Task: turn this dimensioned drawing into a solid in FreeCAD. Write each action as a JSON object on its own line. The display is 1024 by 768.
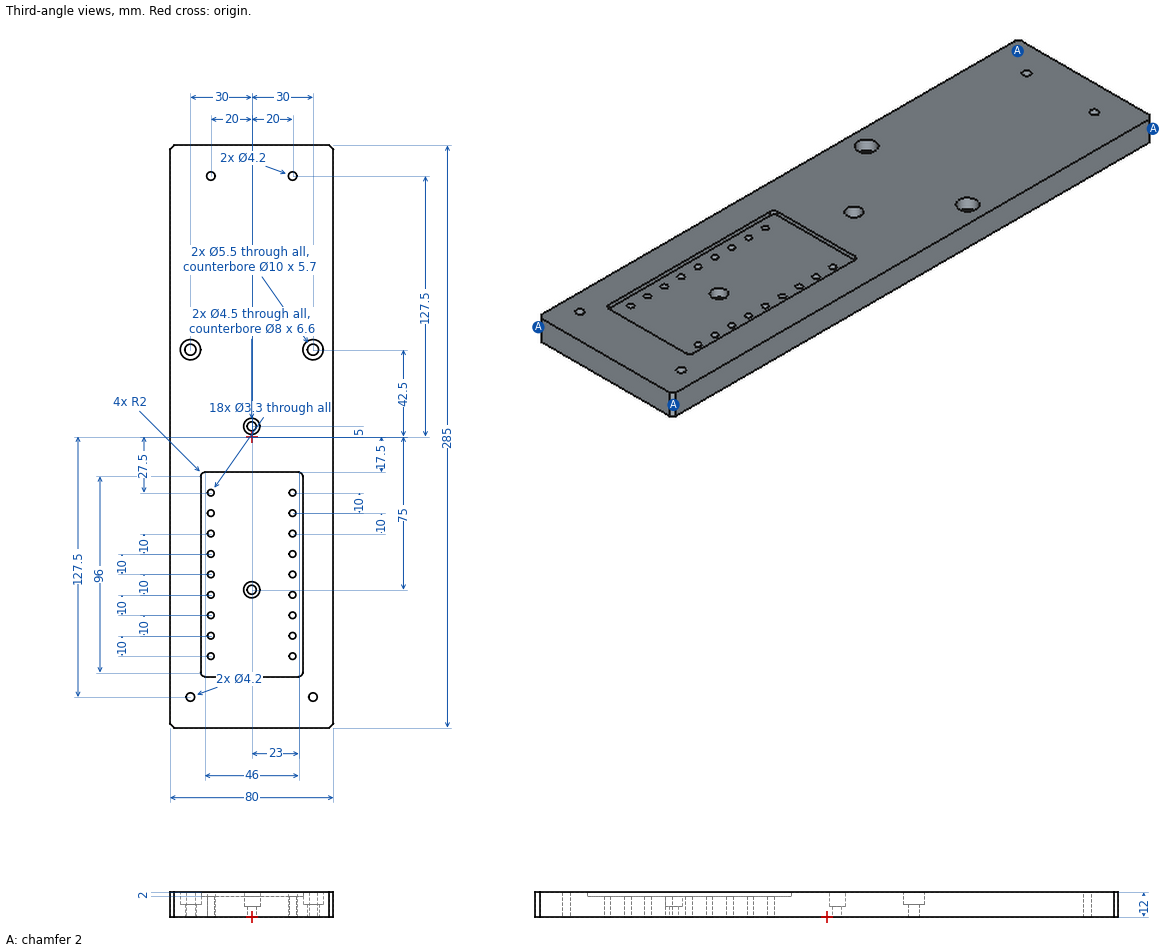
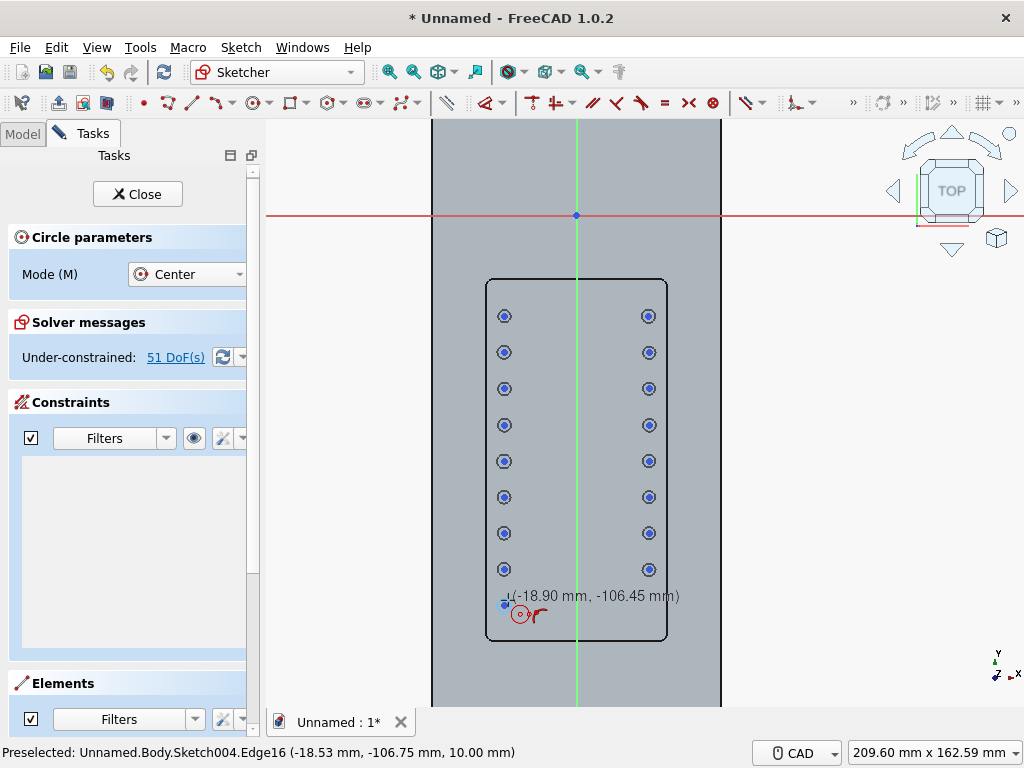
{"action": "scroll", "coordinate": [649, 605], "scroll_direction": "up", "scroll_amount": 7}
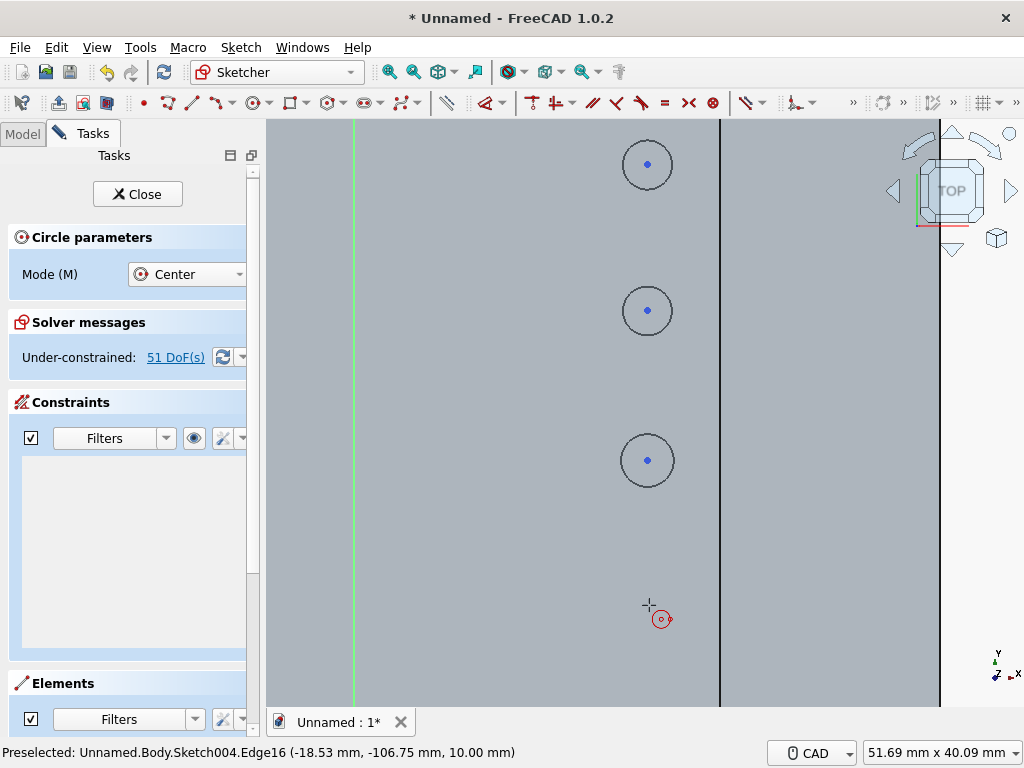
{"action": "scroll", "coordinate": [649, 605], "scroll_direction": "down", "scroll_amount": 7}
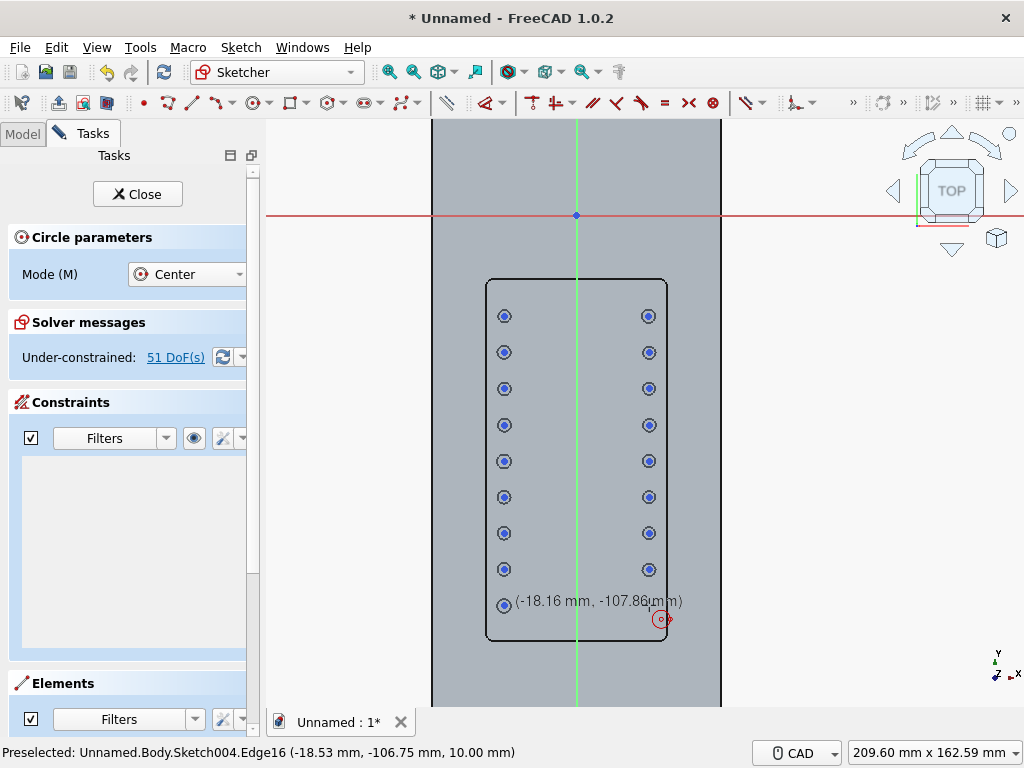
{"action": "left_click", "coordinate": [649, 605]}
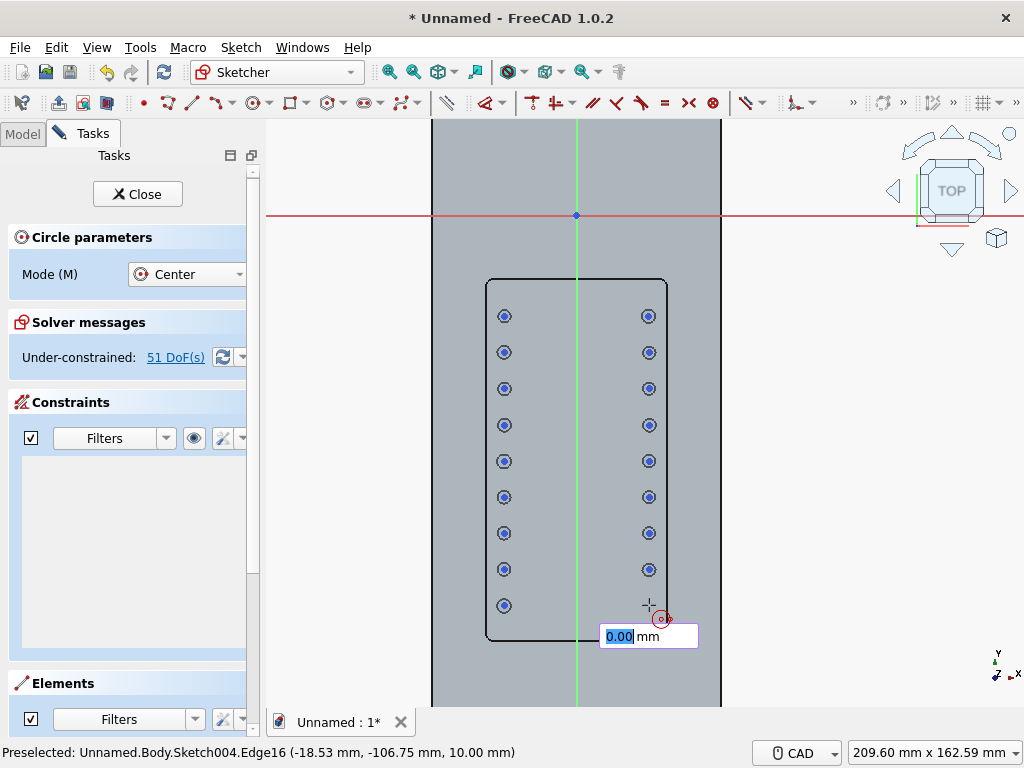
{"action": "scroll", "coordinate": [653, 600], "scroll_direction": "up", "scroll_amount": 5}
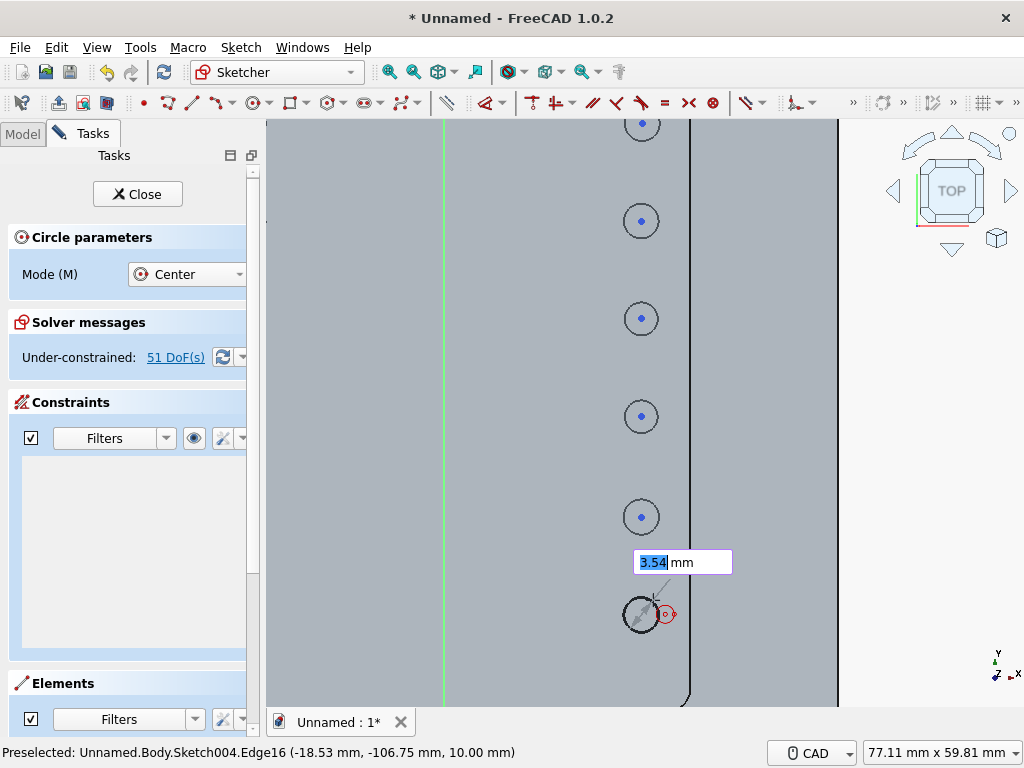
{"action": "left_click", "coordinate": [652, 600]}
{"action": "key", "text": "Escape"}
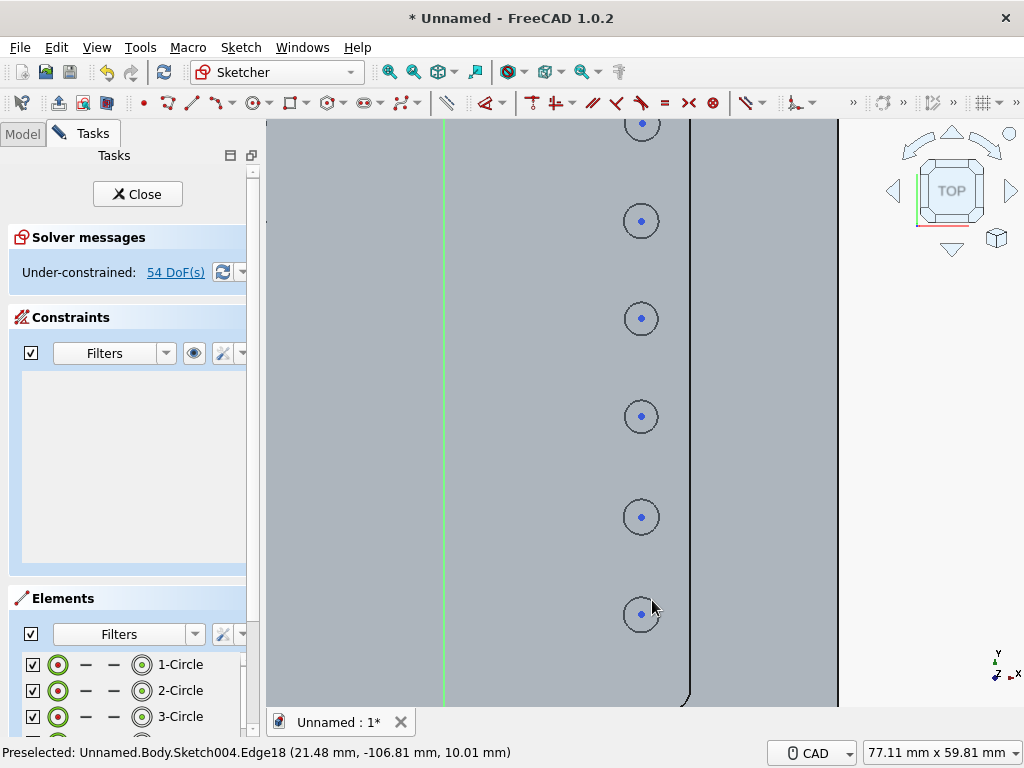
{"action": "scroll", "coordinate": [653, 600], "scroll_direction": "down", "scroll_amount": 5}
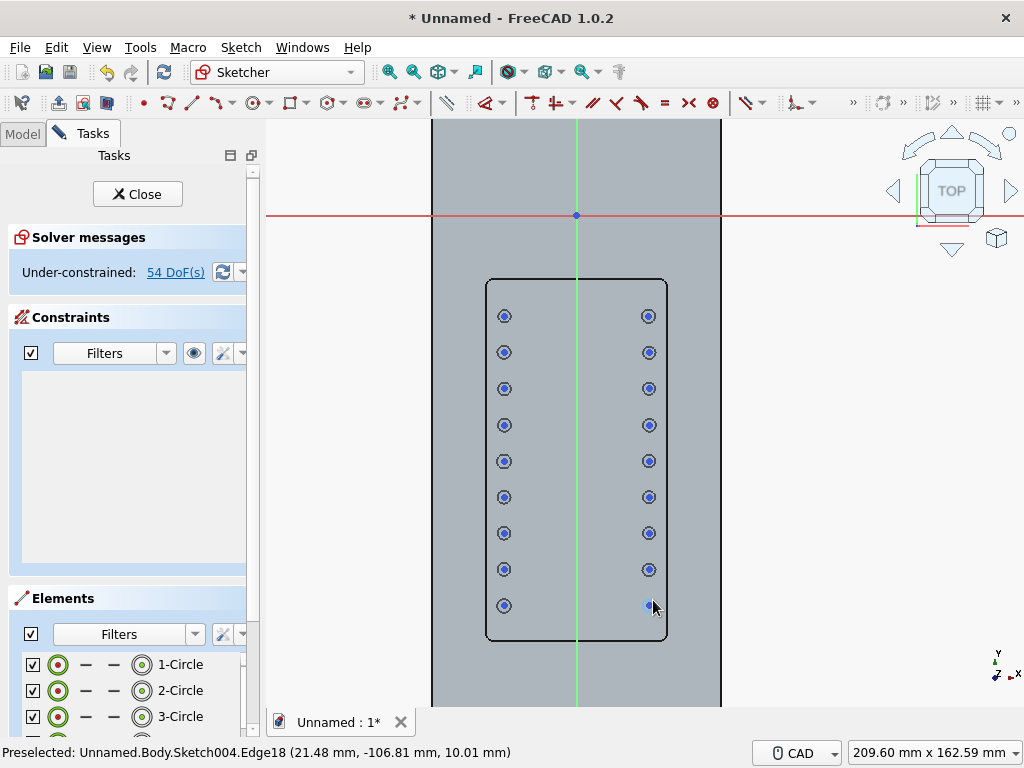
{"action": "scroll", "coordinate": [509, 312], "scroll_direction": "up", "scroll_amount": 5}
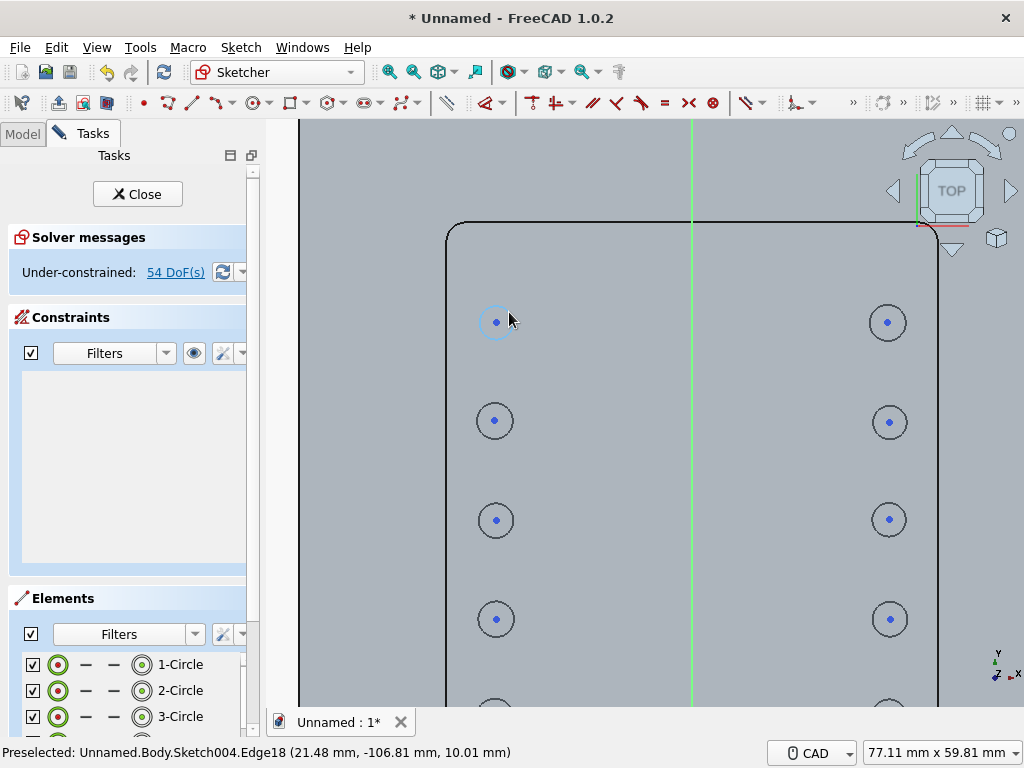
{"action": "left_click", "coordinate": [508, 311]}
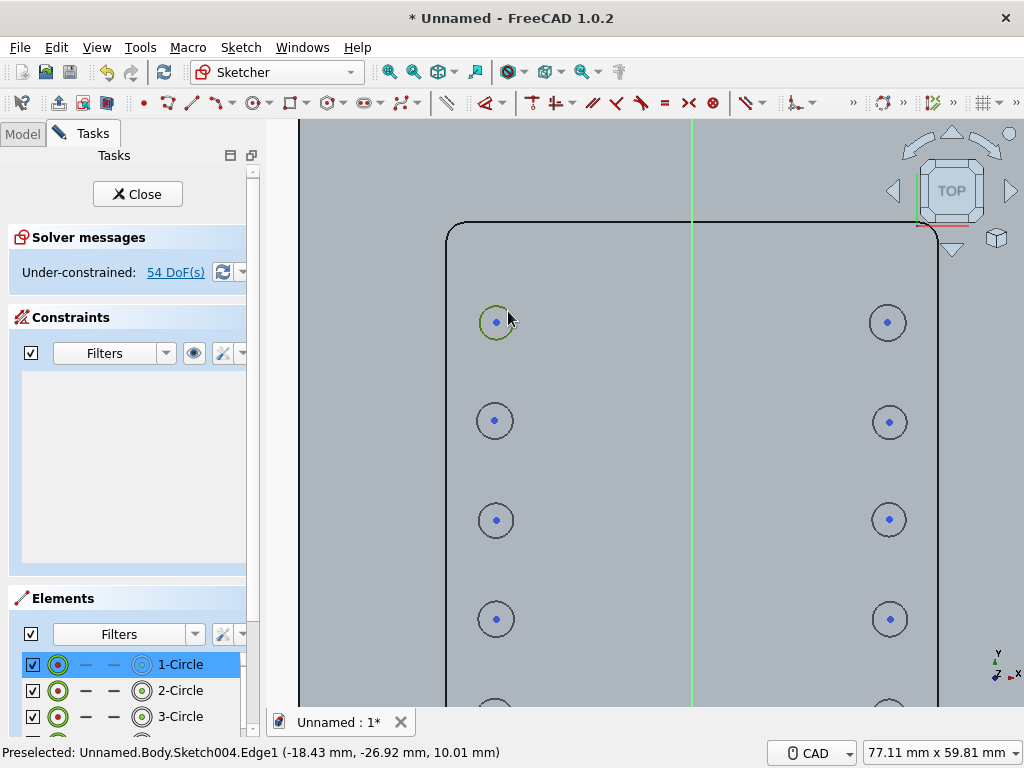
{"action": "scroll", "coordinate": [509, 312], "scroll_direction": "down", "scroll_amount": 5}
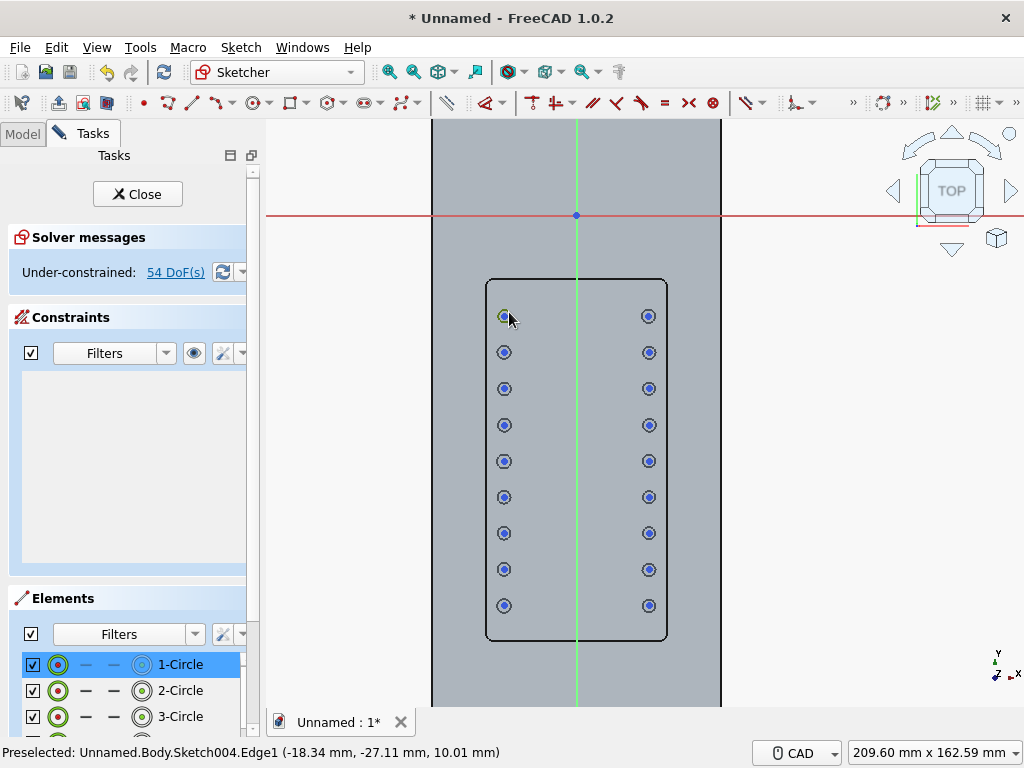
{"action": "scroll", "coordinate": [653, 312], "scroll_direction": "up", "scroll_amount": 4}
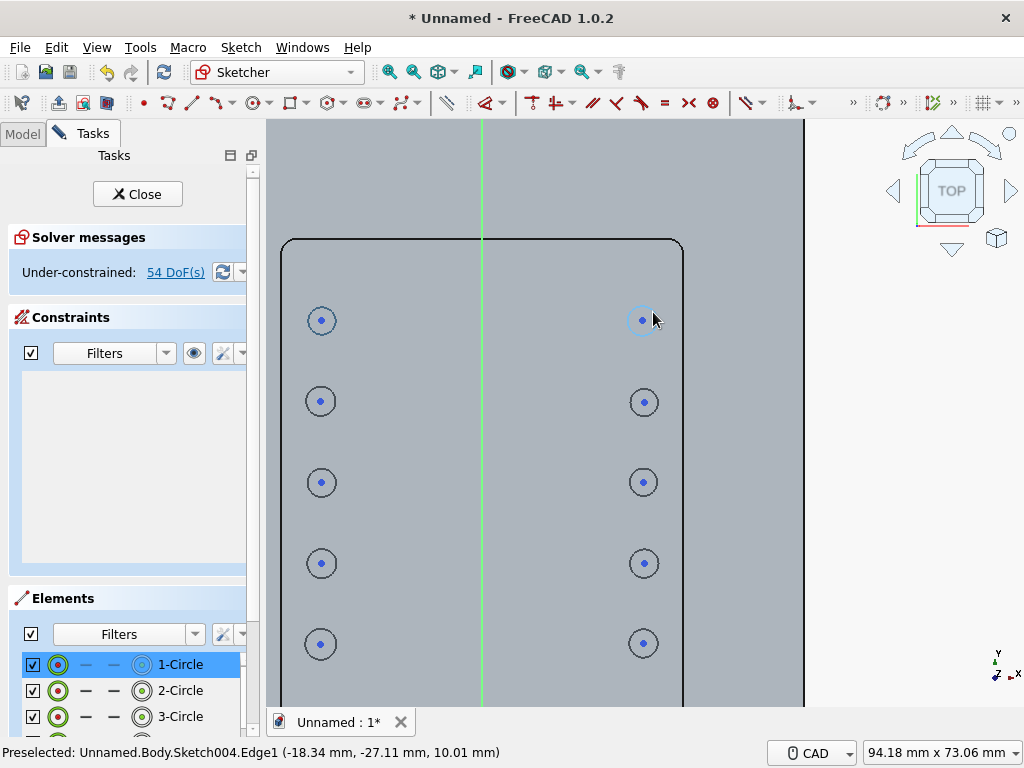
{"action": "left_click", "coordinate": [653, 311]}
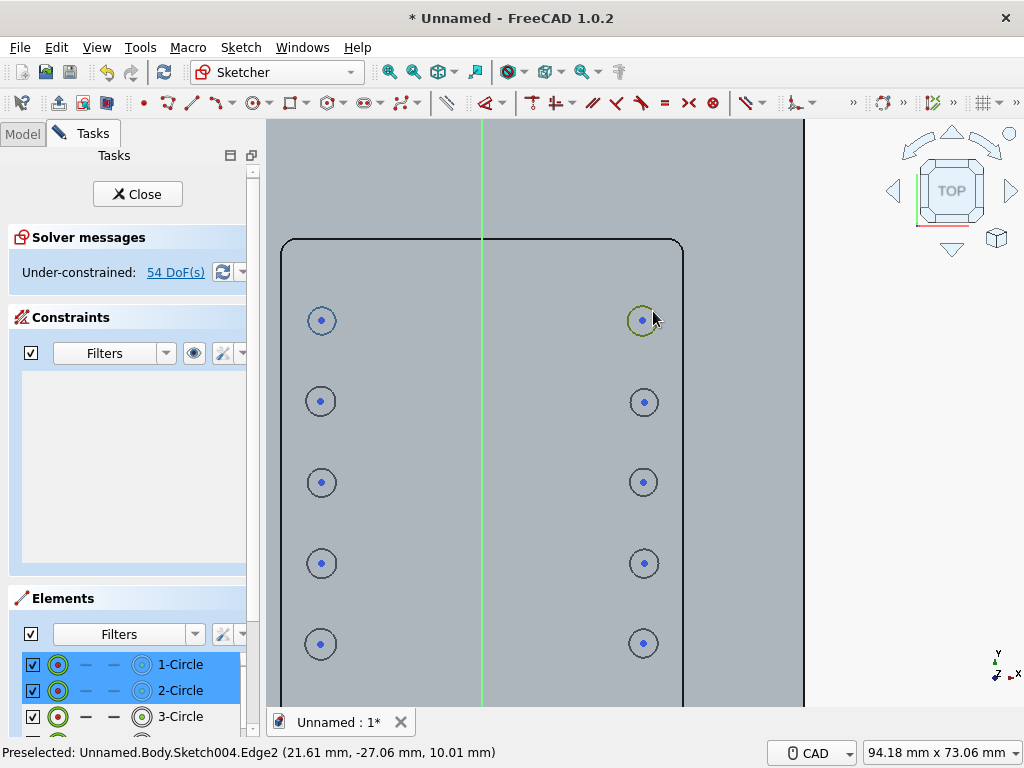
{"action": "left_click", "coordinate": [654, 393]}